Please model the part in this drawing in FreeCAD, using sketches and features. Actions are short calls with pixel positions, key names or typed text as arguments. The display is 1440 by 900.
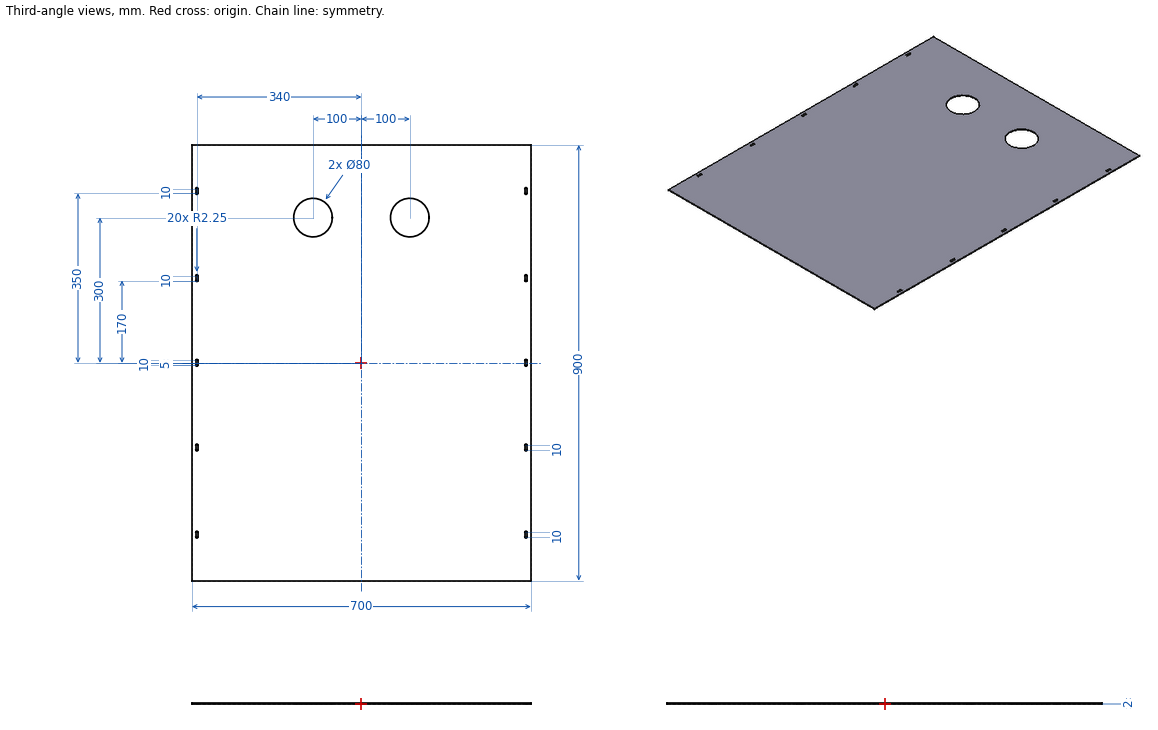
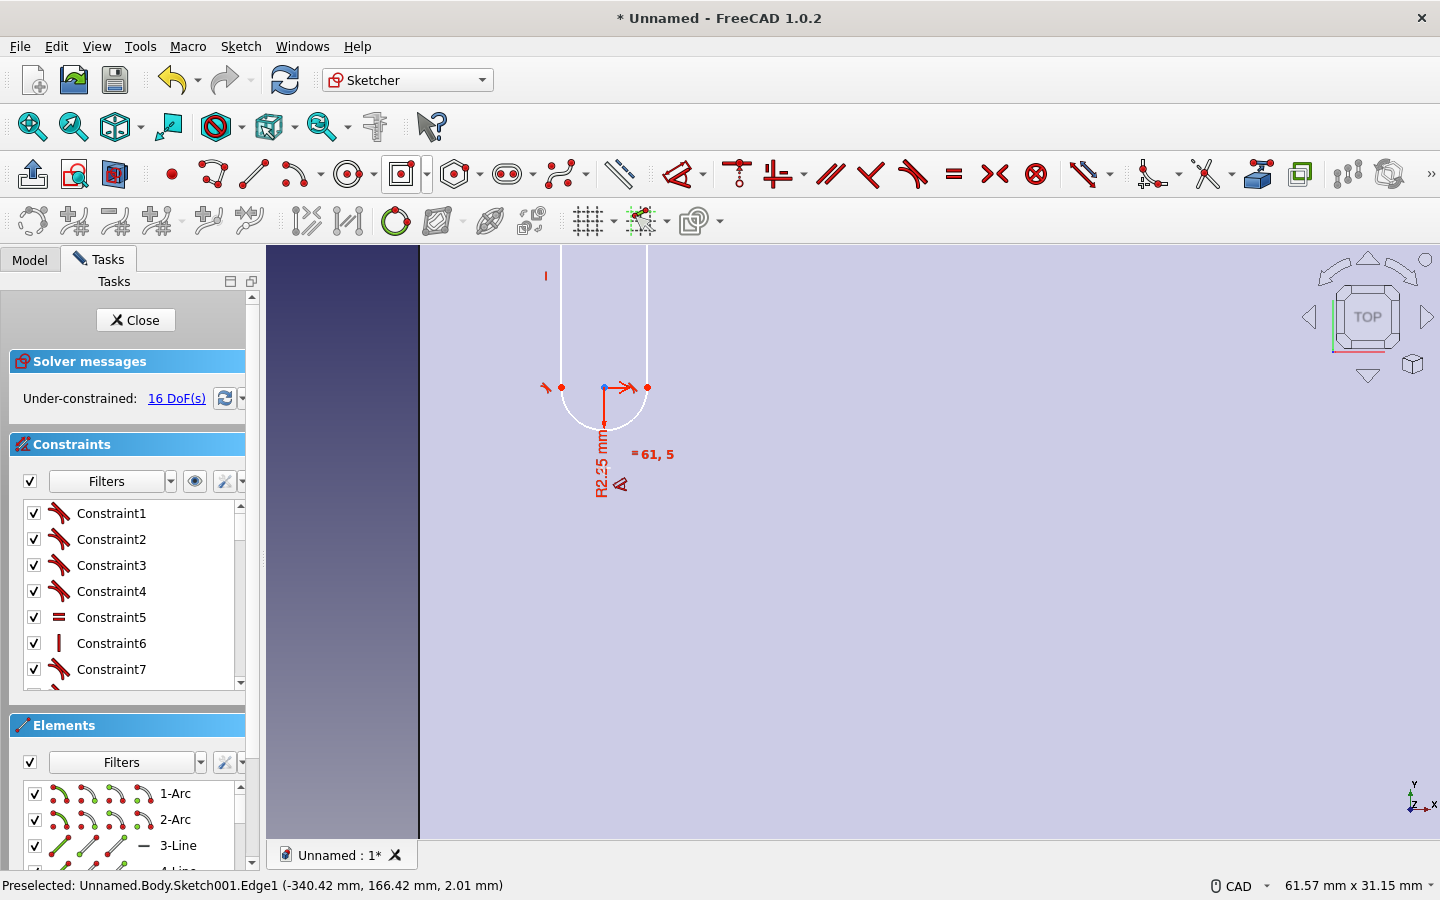
scroll(567, 436, down, 17)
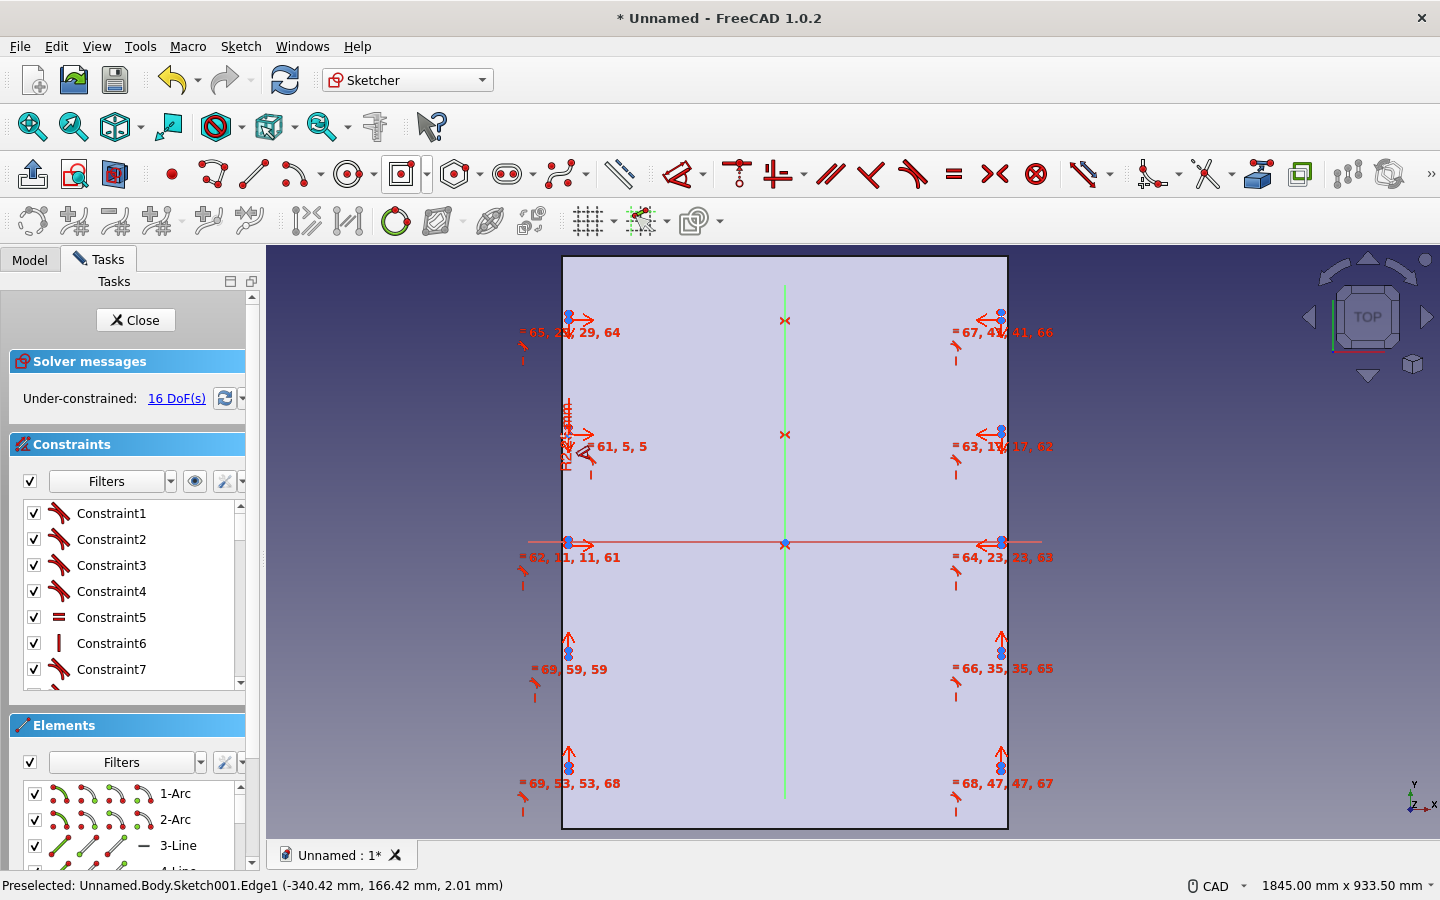
scroll(567, 432, up, 10)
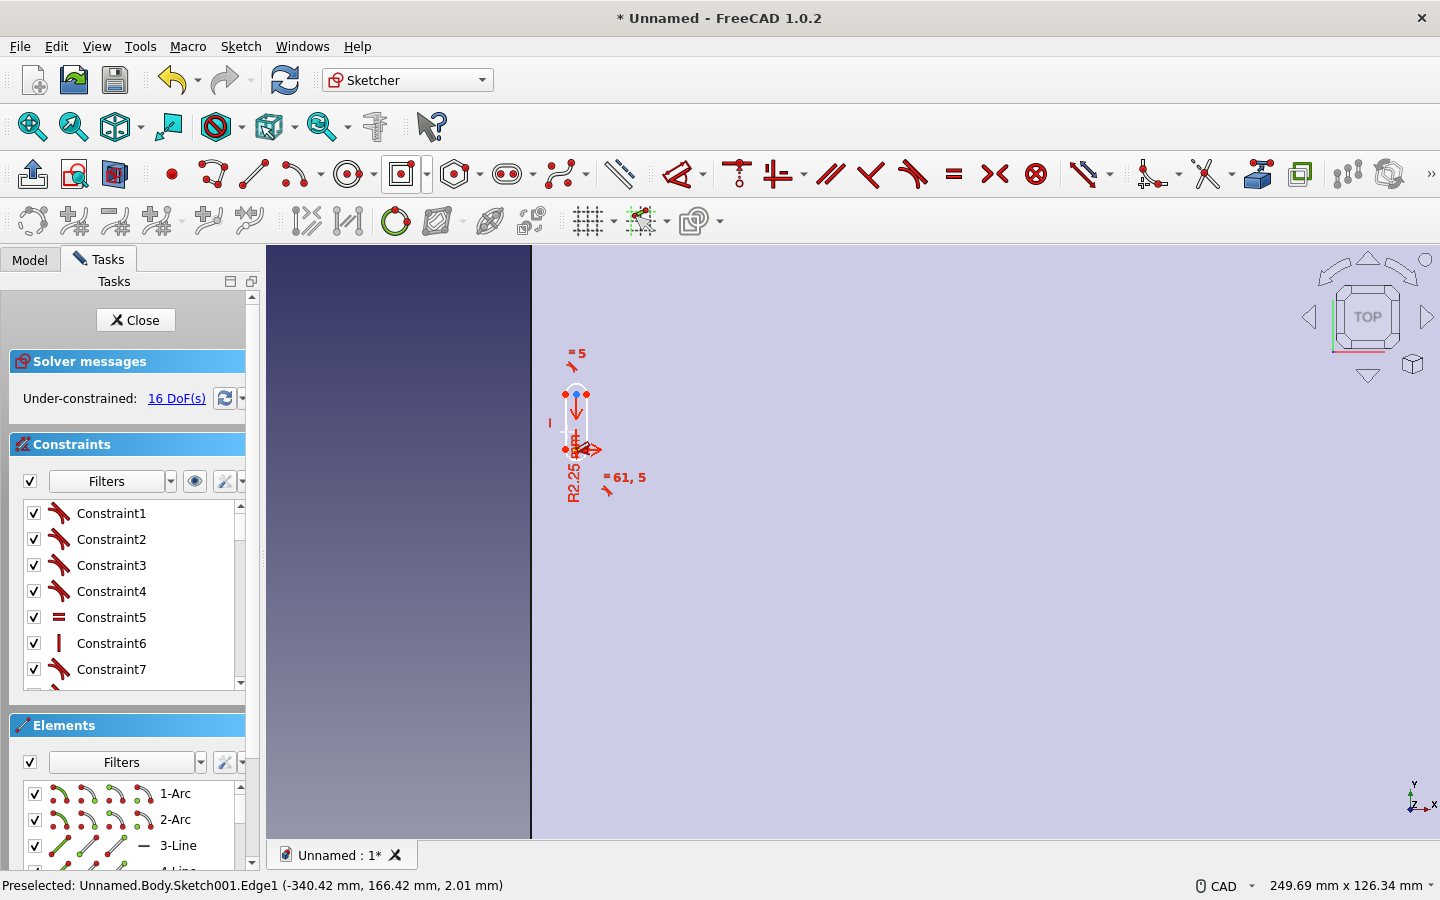
click(566, 433)
click(532, 422)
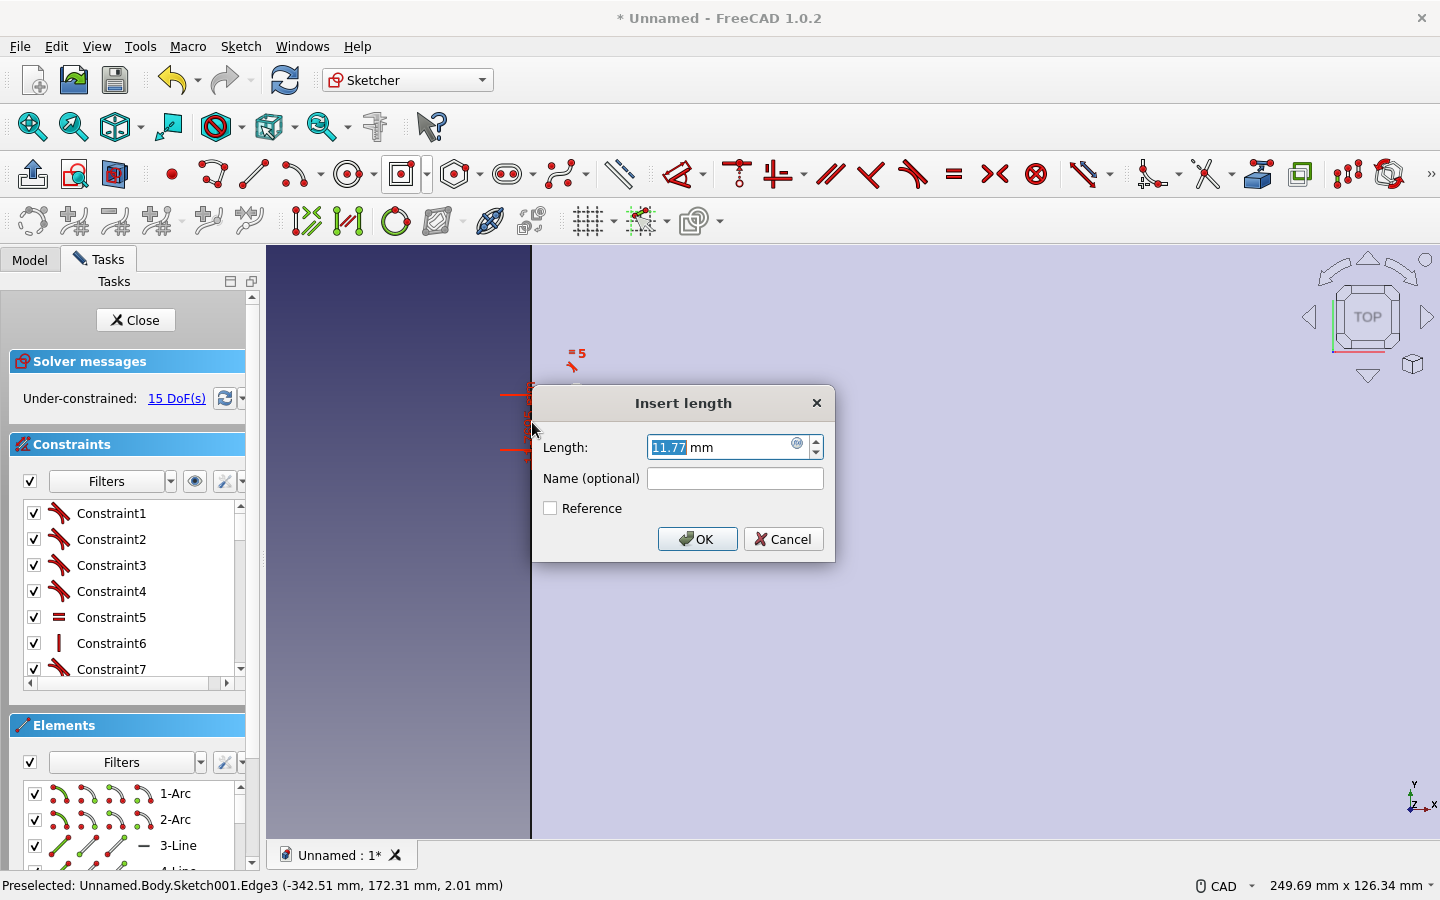
text(10)
key(Return)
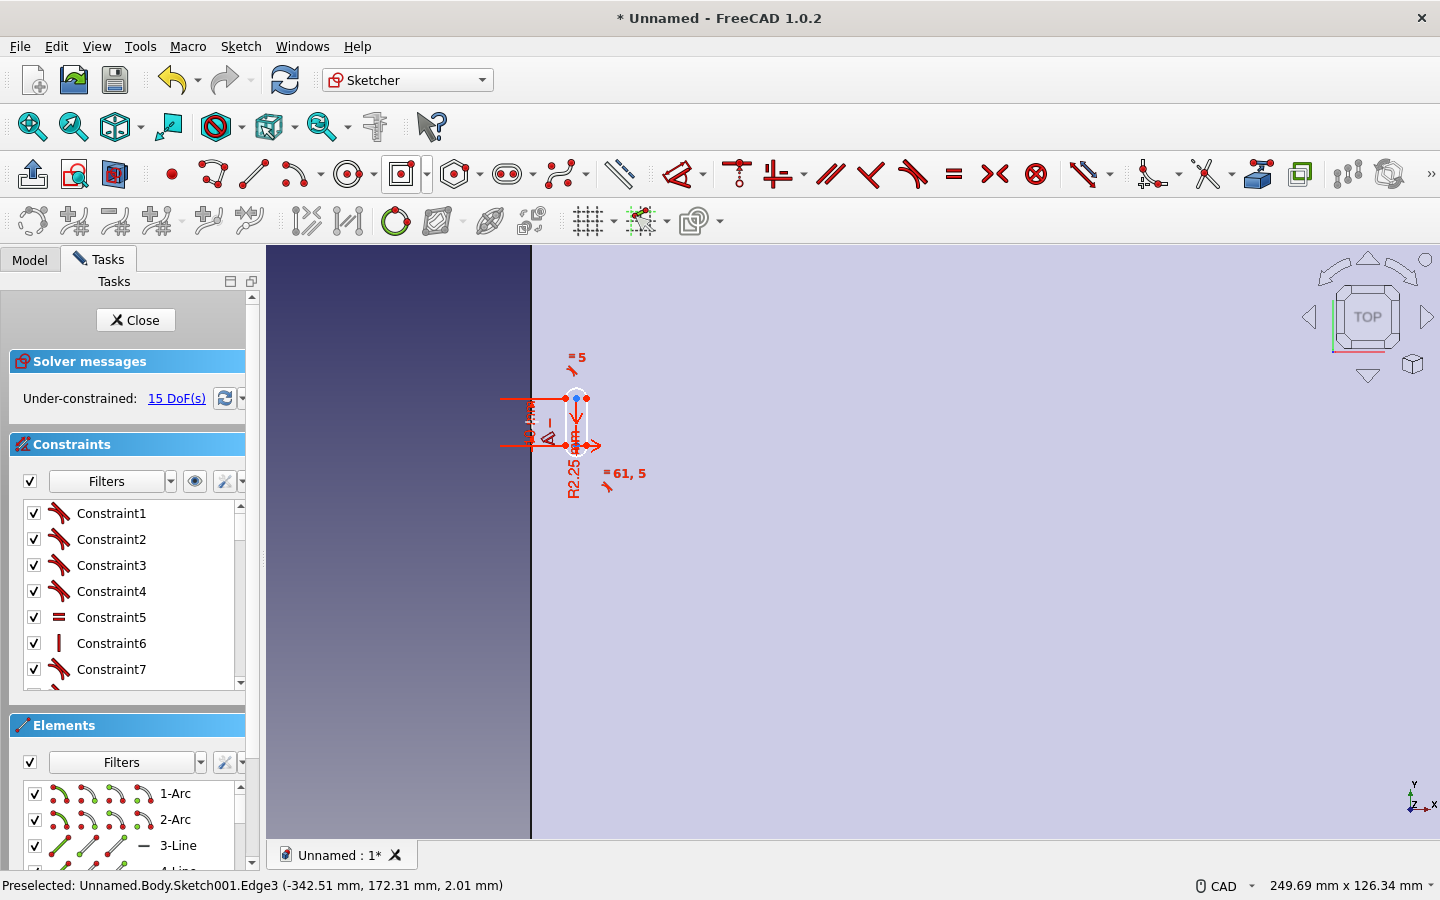
scroll(611, 455, down, 11)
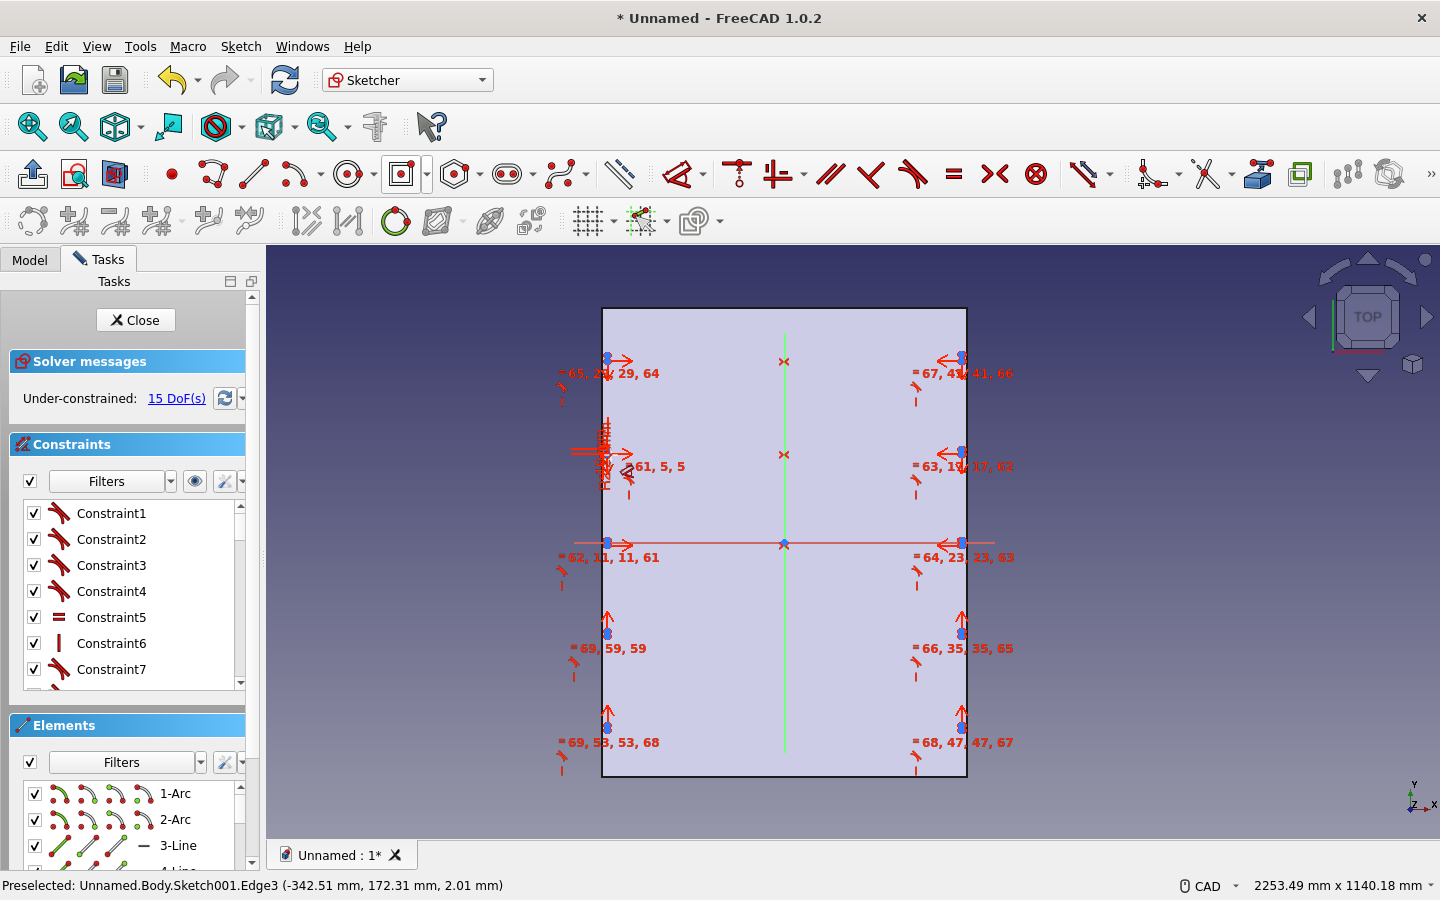
scroll(606, 544, up, 13)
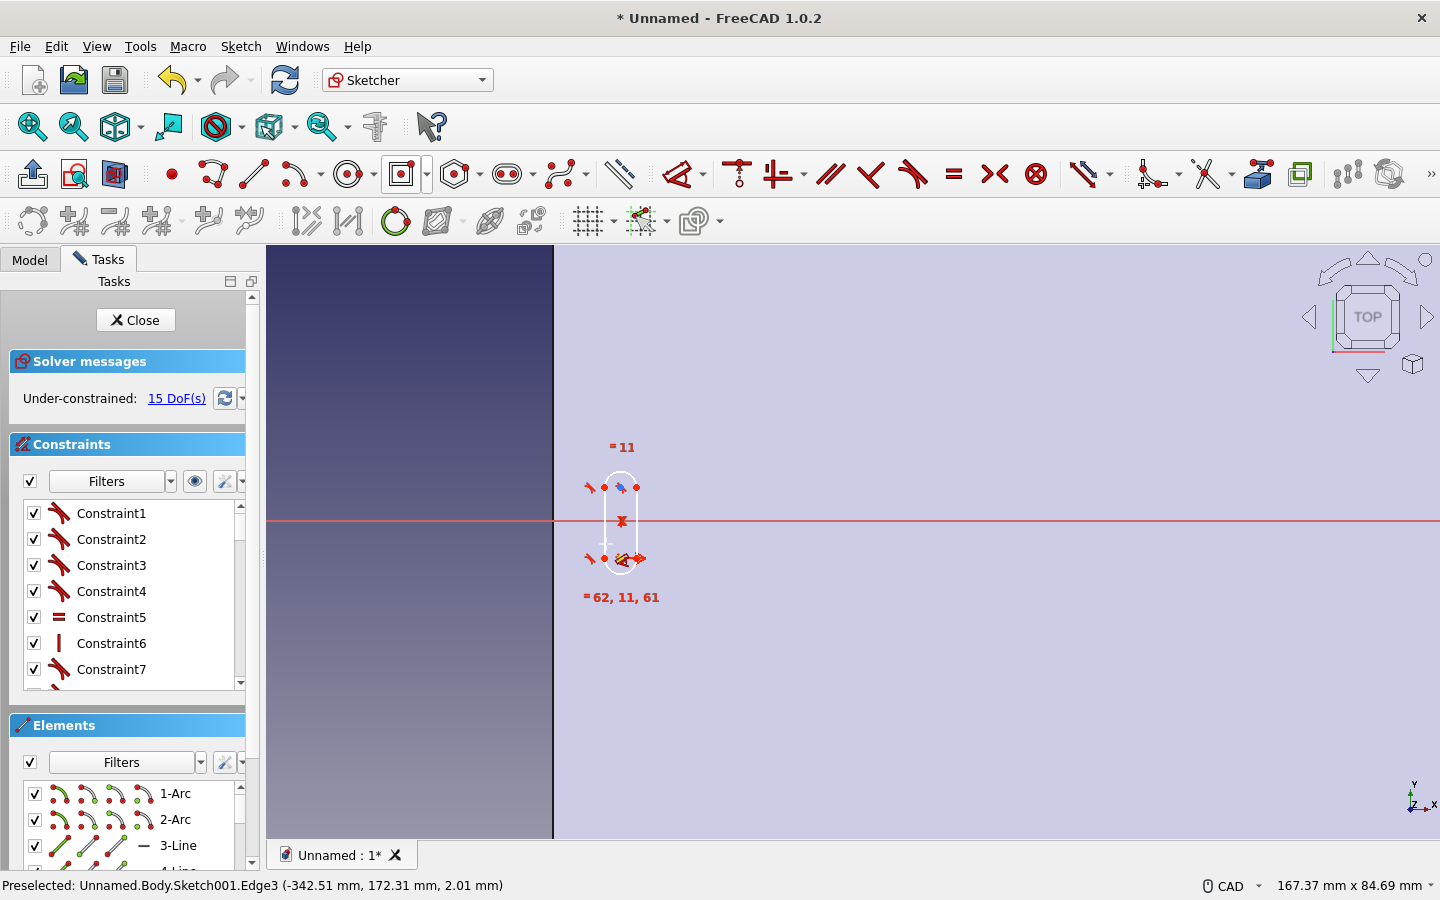
click(605, 537)
click(571, 507)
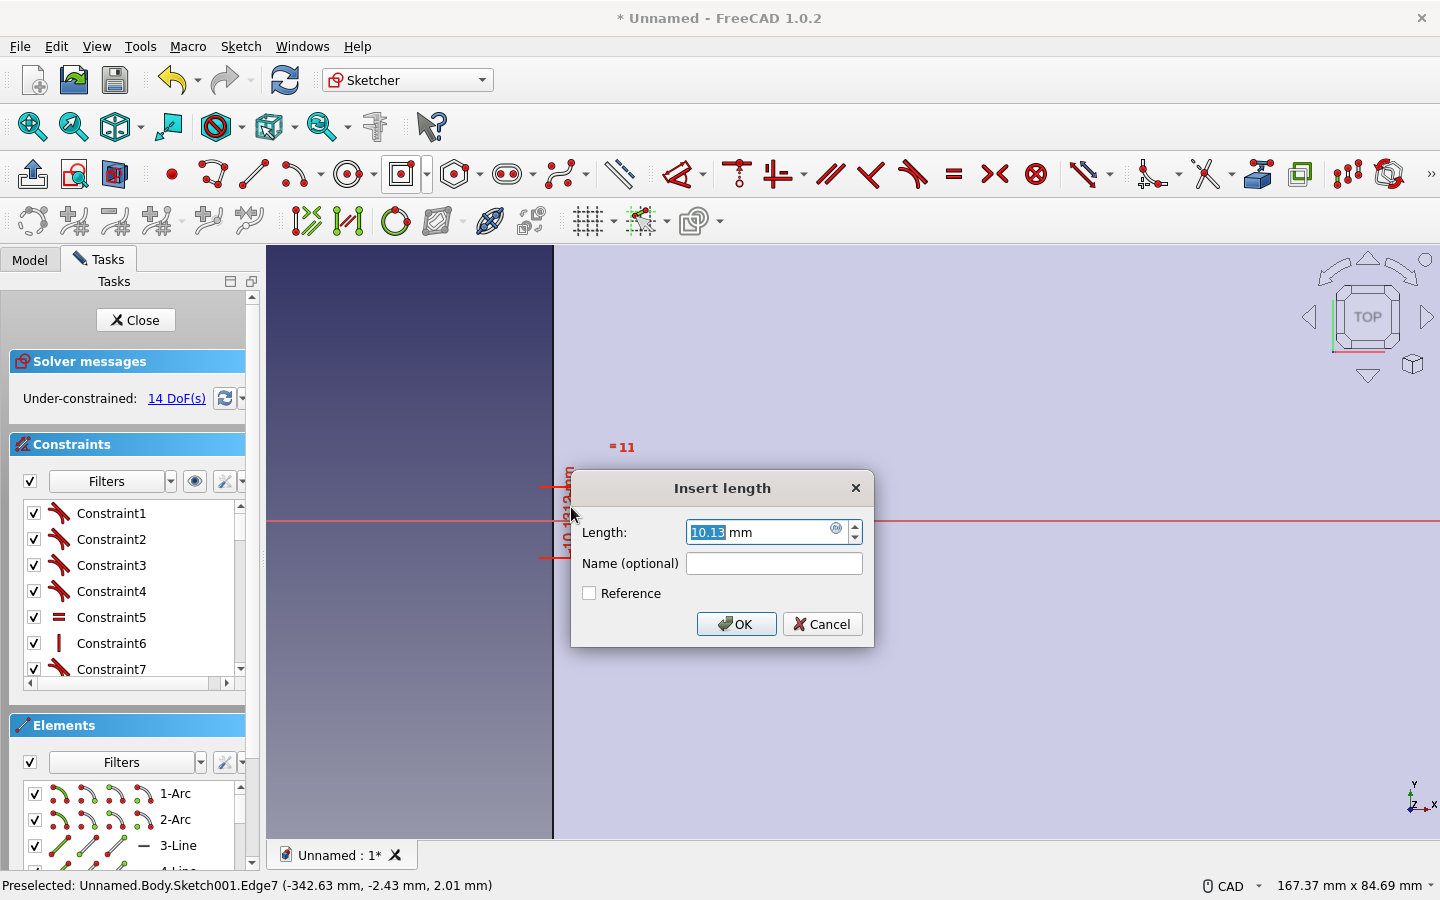
text(10)
key(Return)